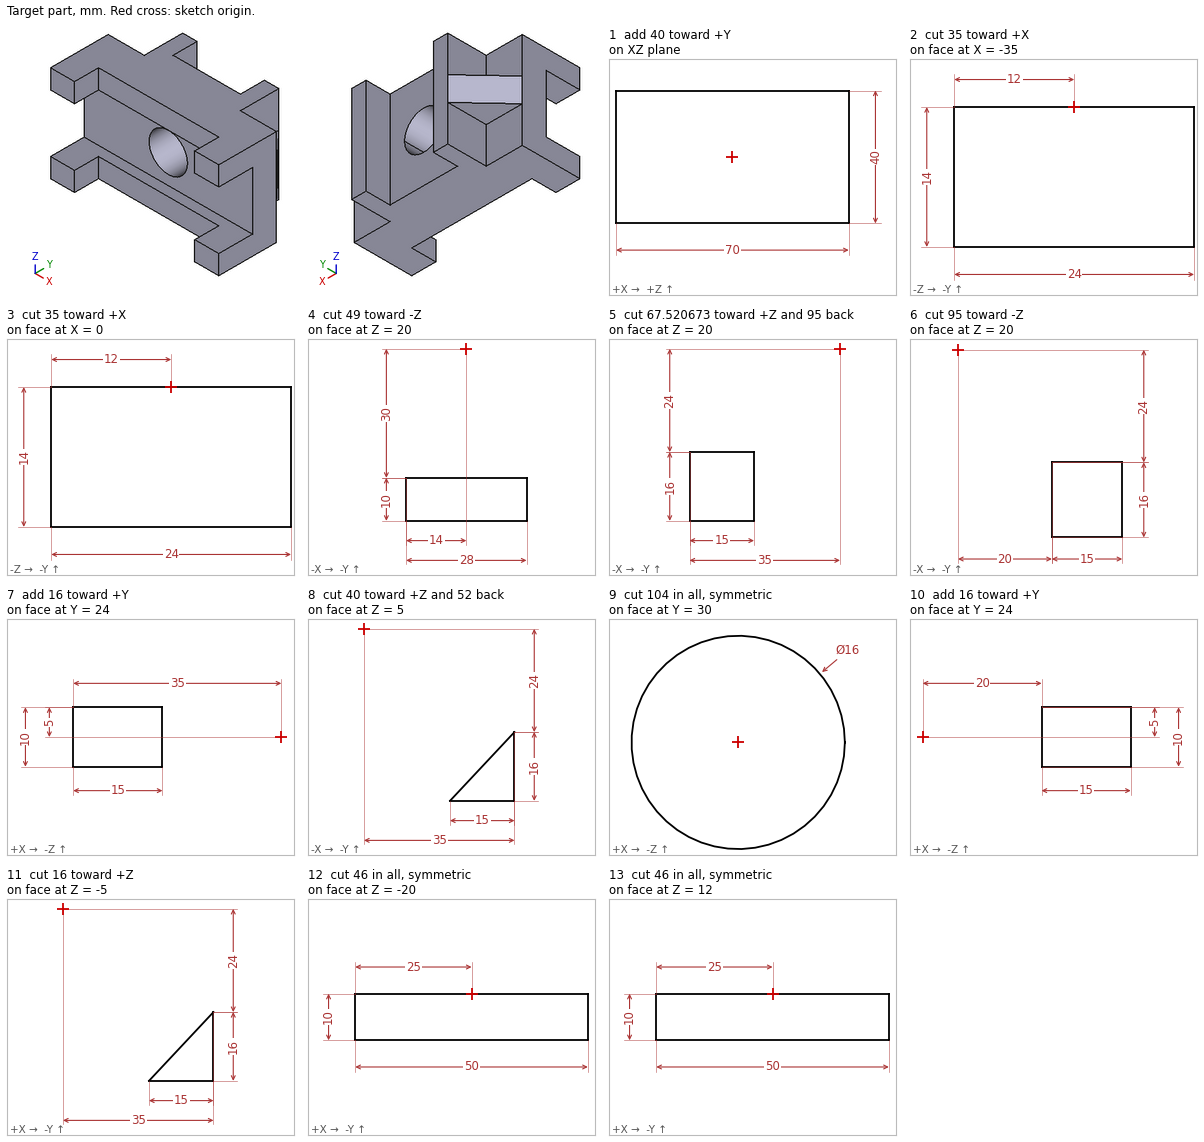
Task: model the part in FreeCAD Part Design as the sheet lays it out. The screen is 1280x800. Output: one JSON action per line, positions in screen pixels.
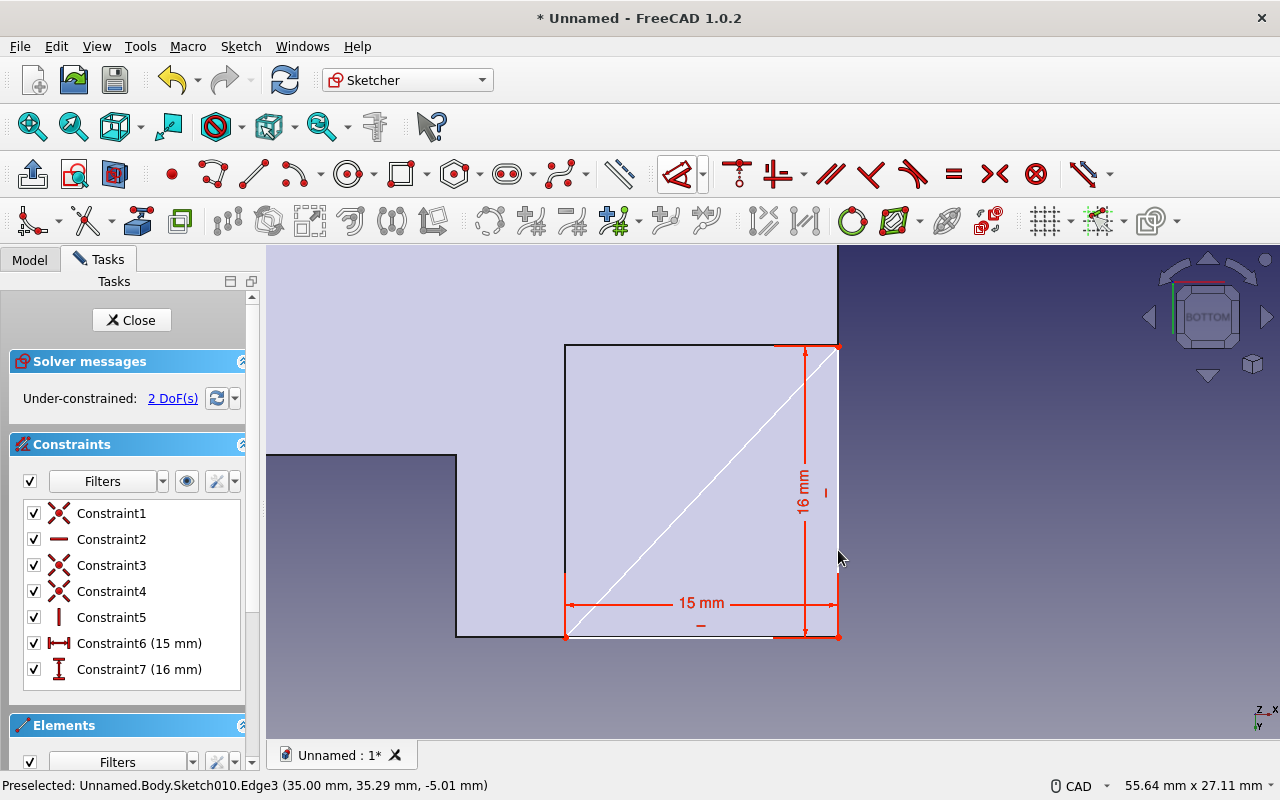
{"action": "left_click", "coordinate": [838, 346]}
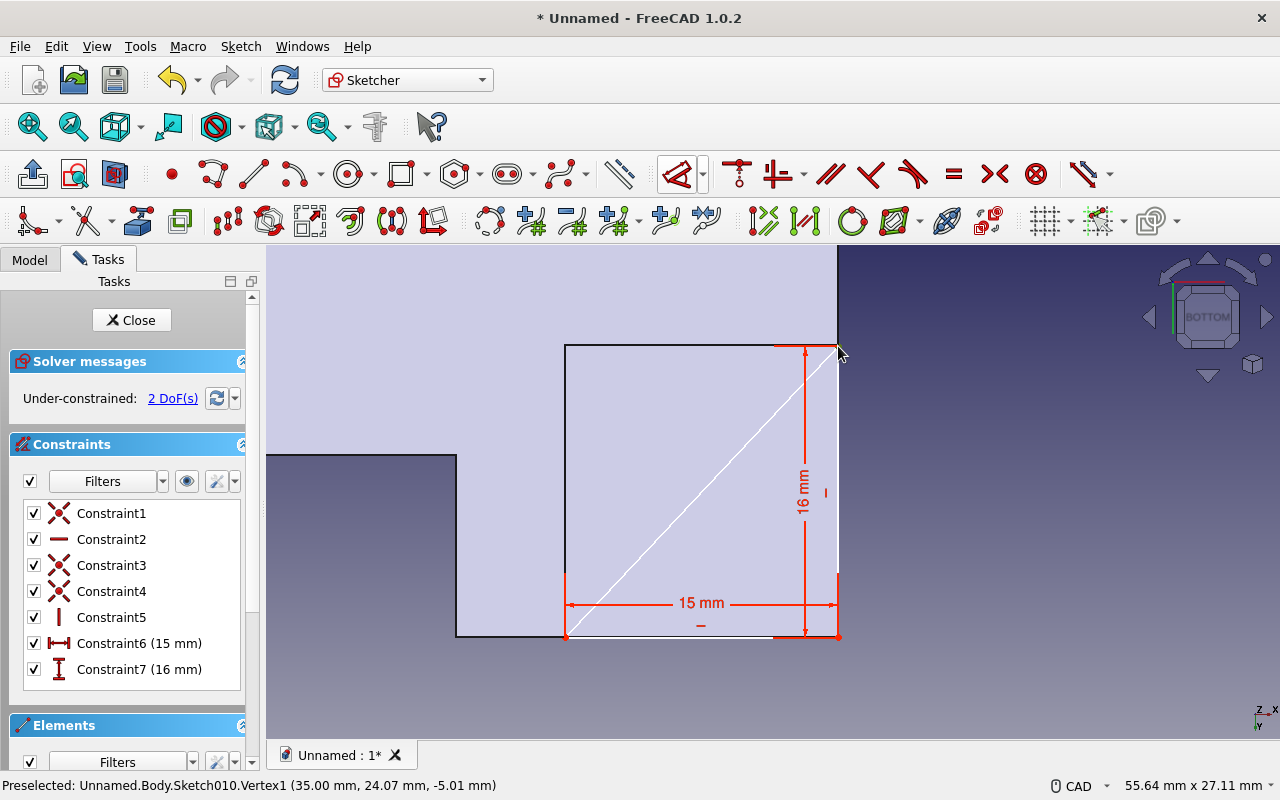
{"action": "left_click", "coordinate": [702, 174]}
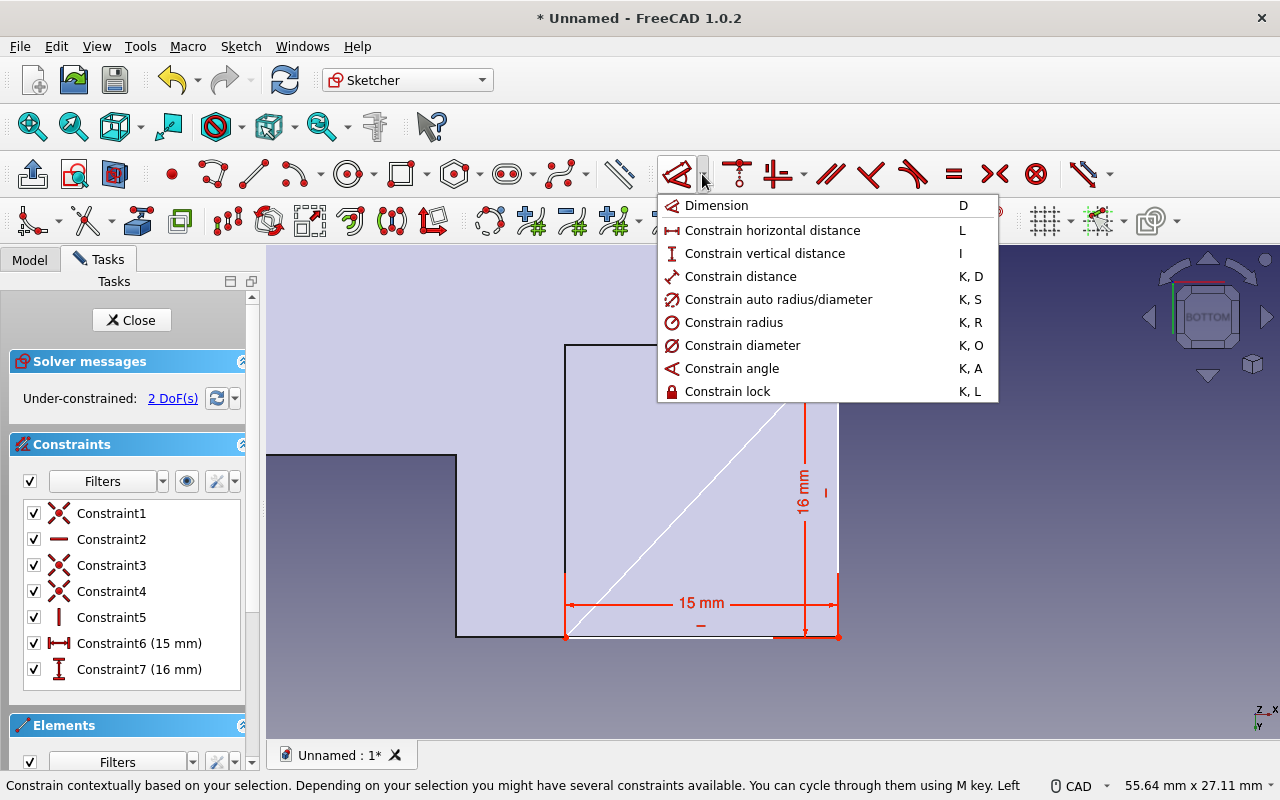
{"action": "left_click", "coordinate": [828, 230]}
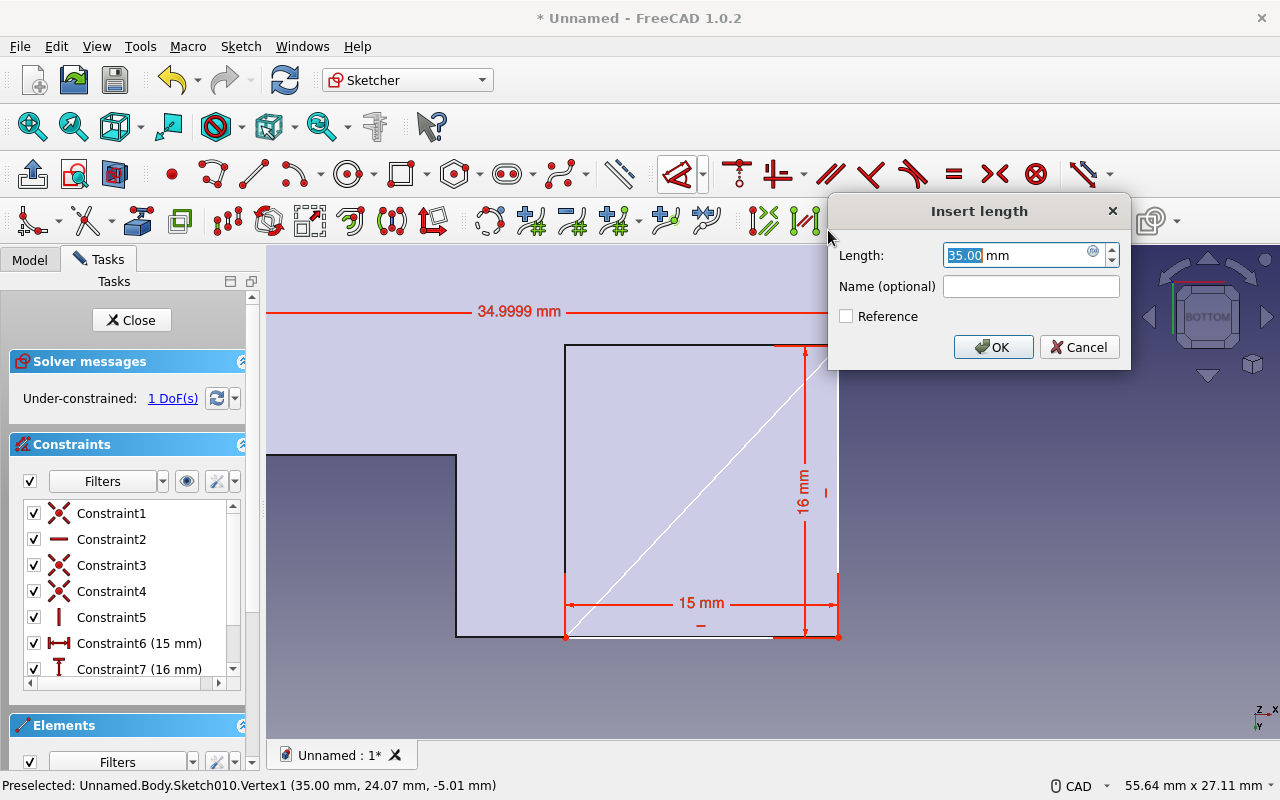
{"action": "type", "text": "35"}
{"action": "key", "text": "Return"}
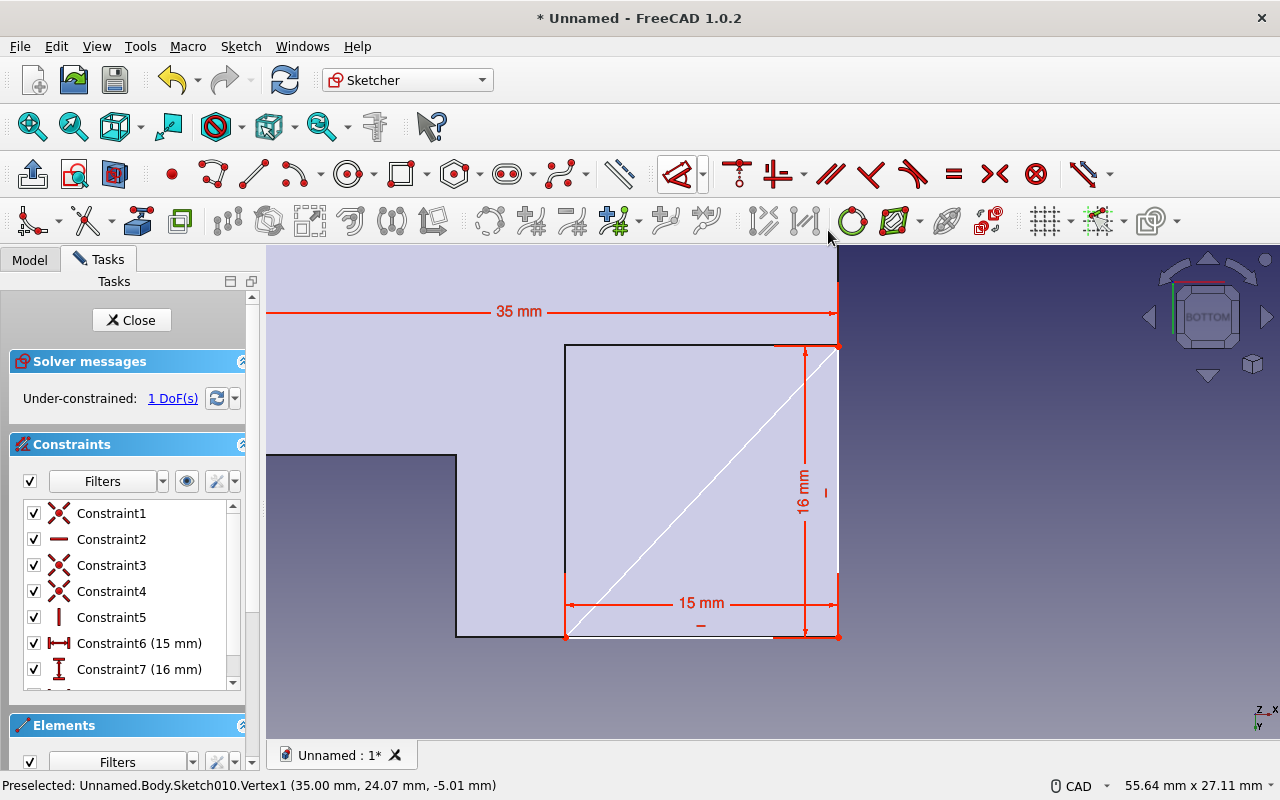
{"action": "left_click", "coordinate": [838, 346]}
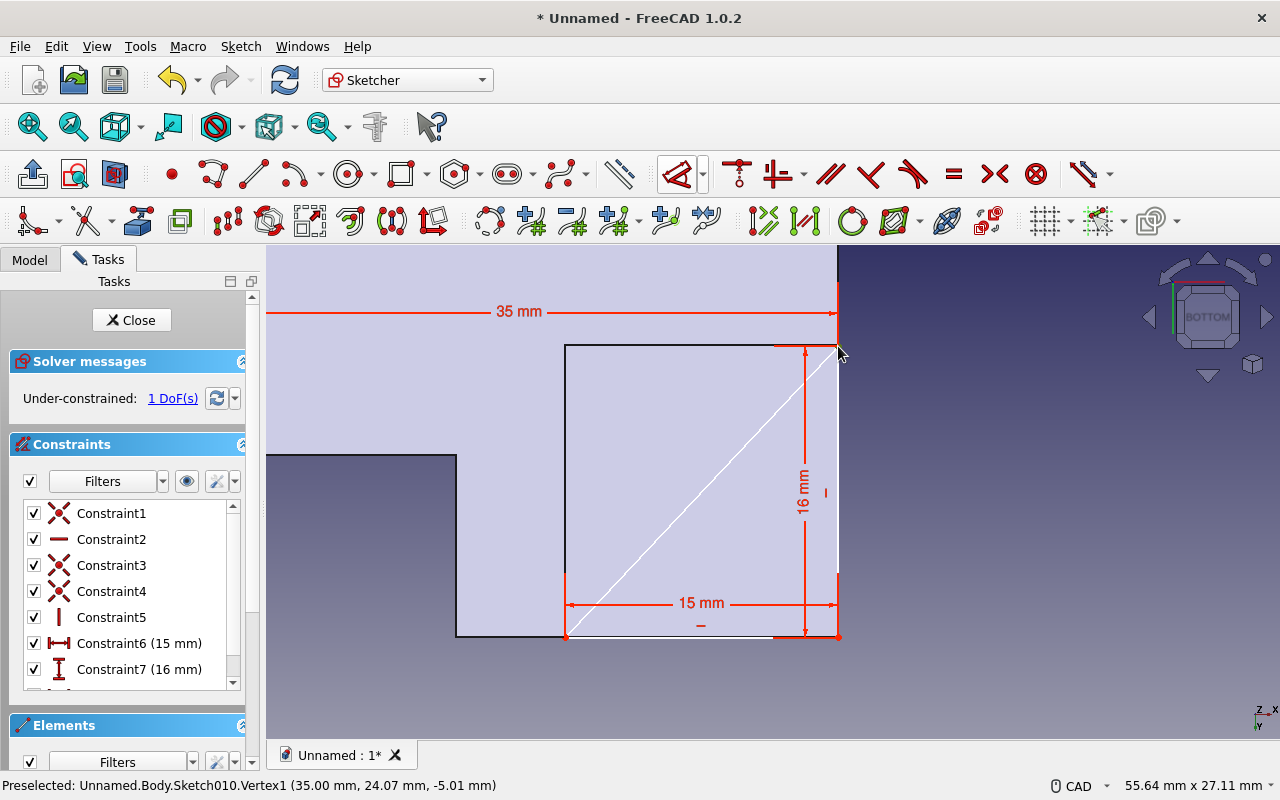
{"action": "key", "text": "i"}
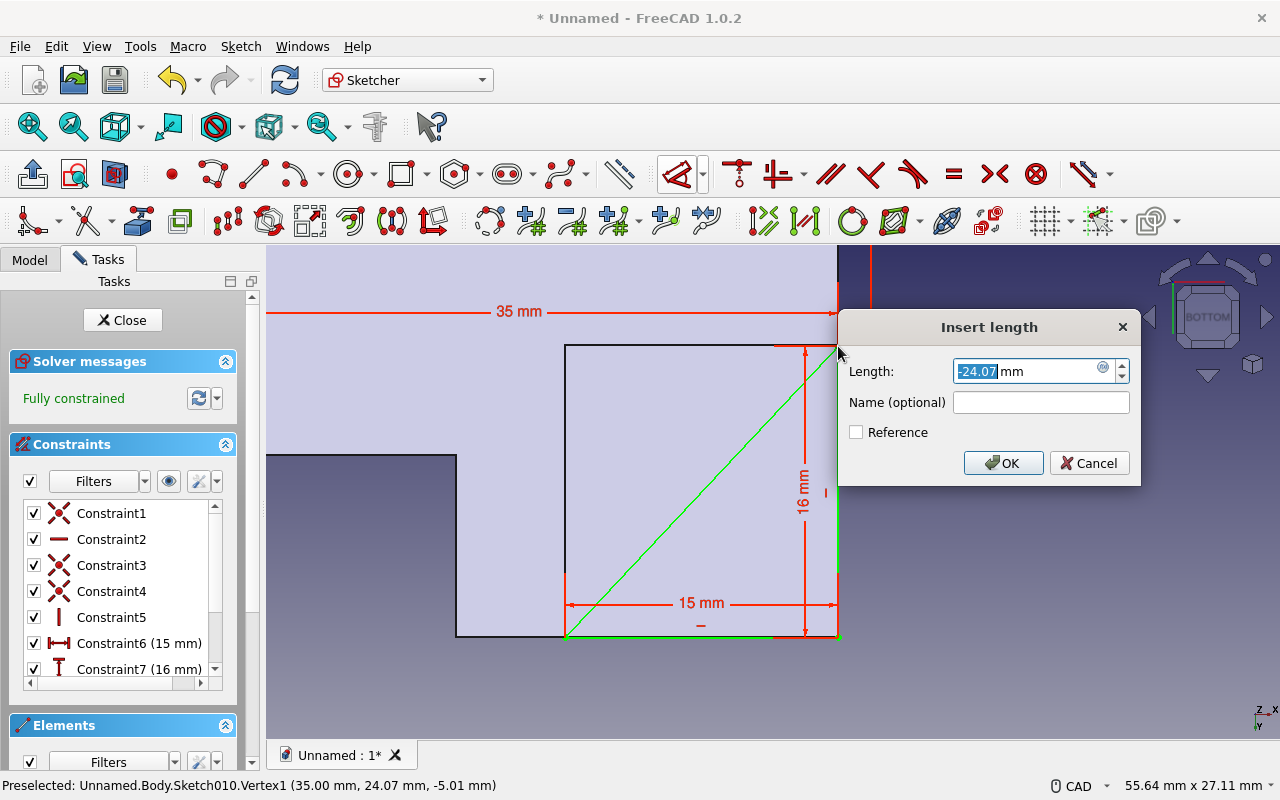
{"action": "type", "text": "-24"}
{"action": "key", "text": "Return"}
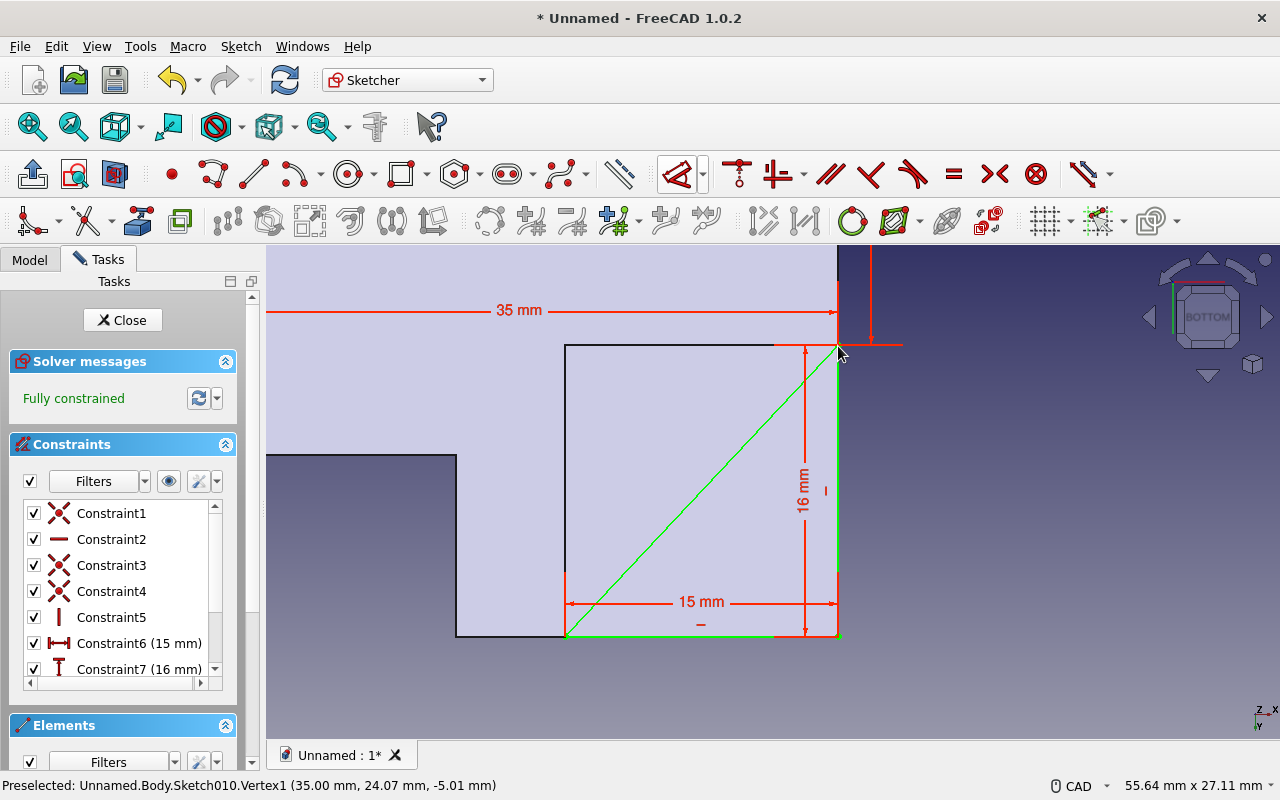
{"action": "left_click", "coordinate": [123, 320]}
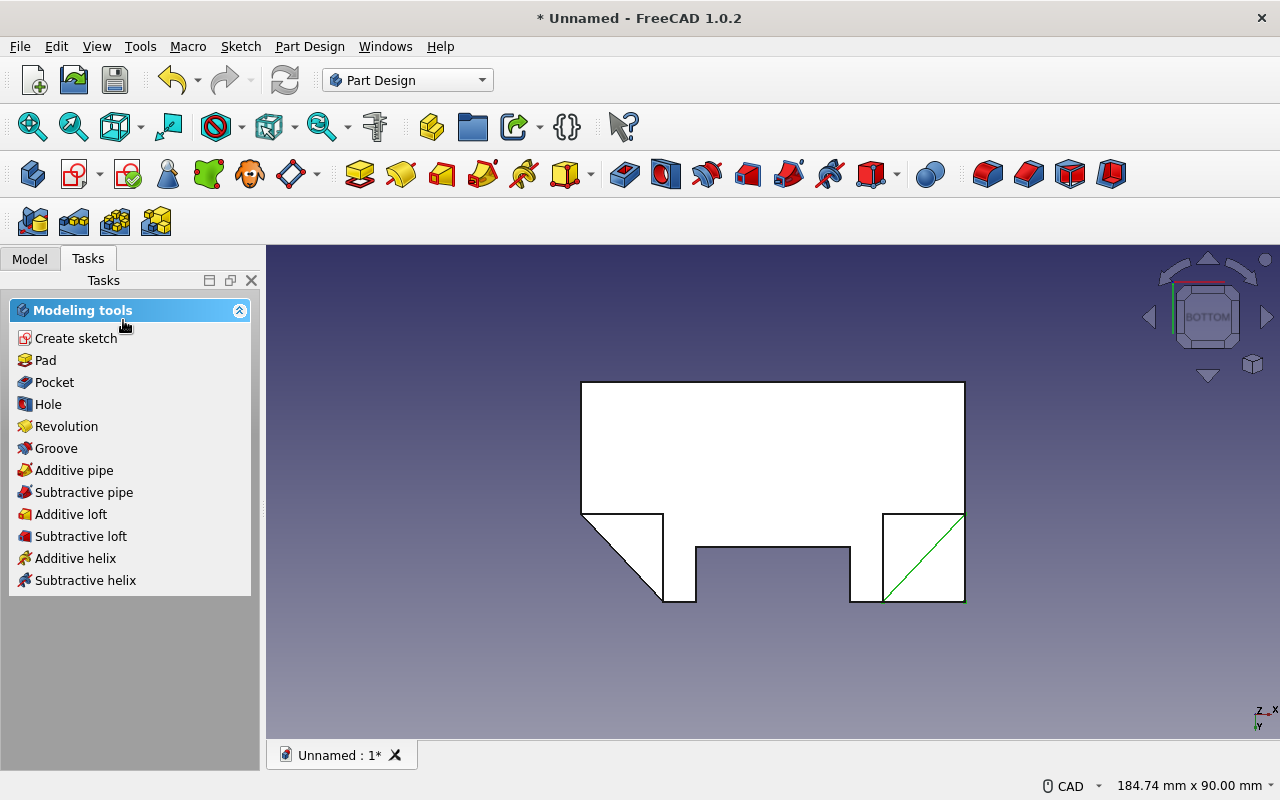
{"action": "left_click", "coordinate": [625, 174]}